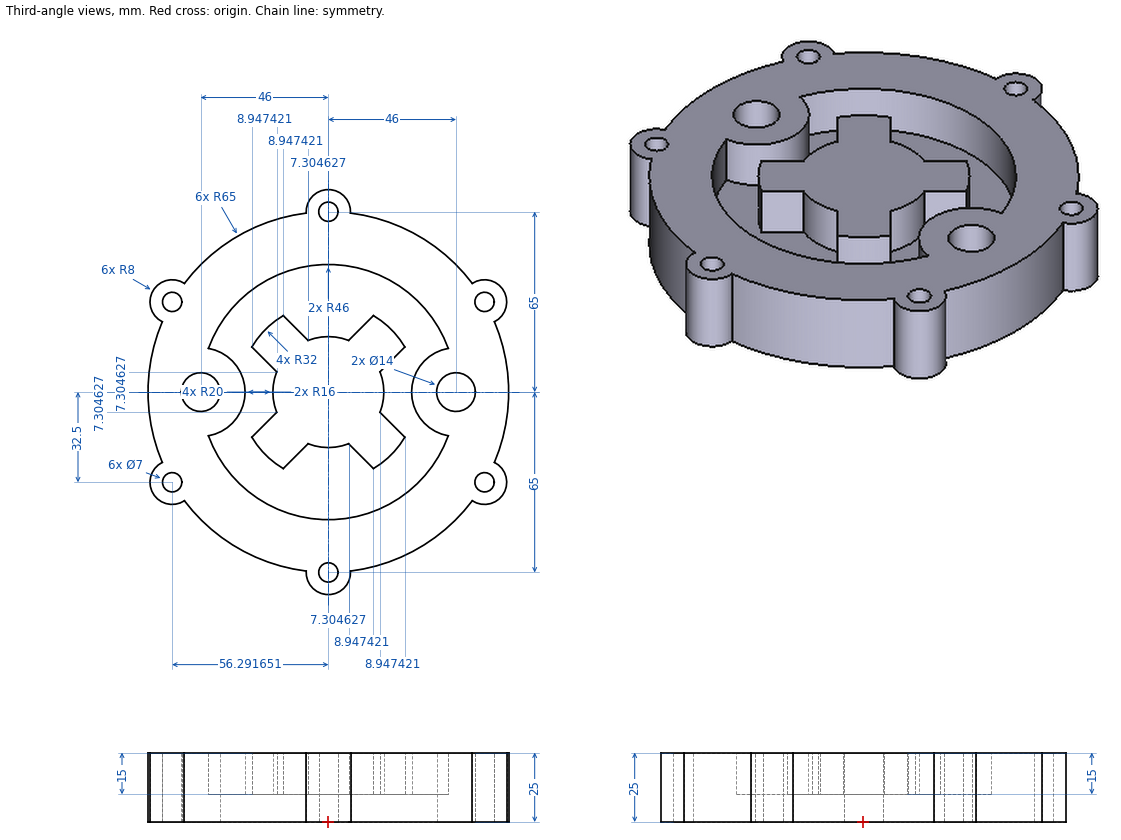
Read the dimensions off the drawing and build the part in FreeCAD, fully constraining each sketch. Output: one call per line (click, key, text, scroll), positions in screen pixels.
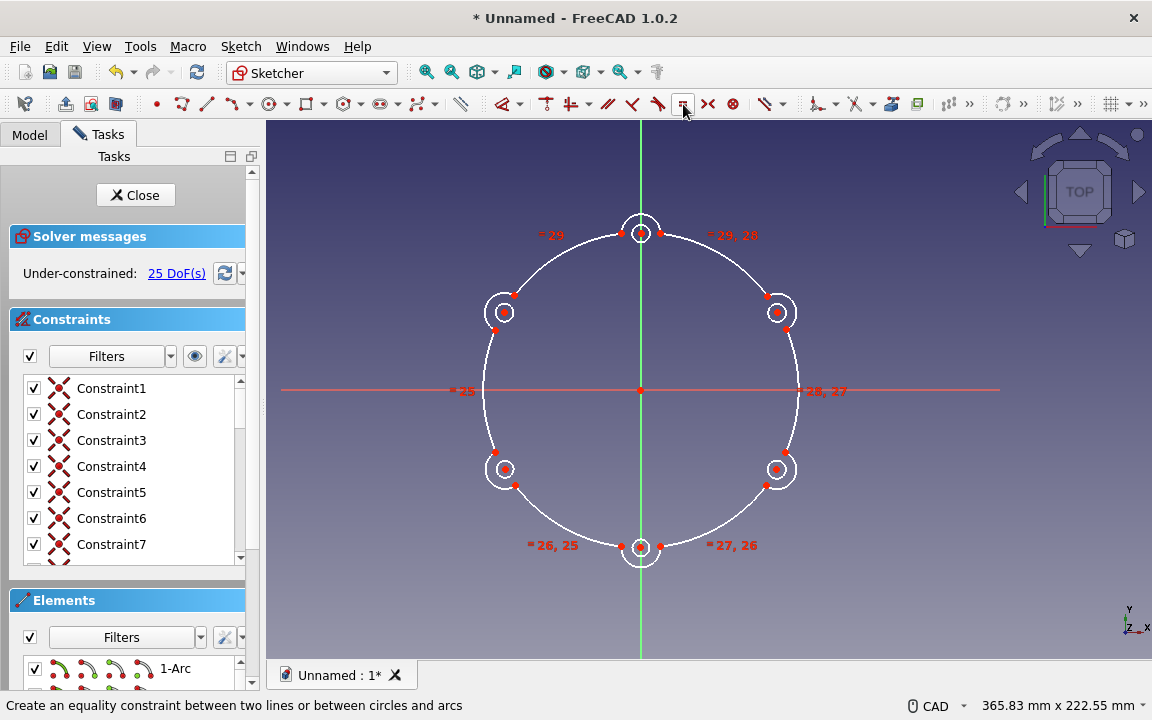
scroll(486, 467, up, 2)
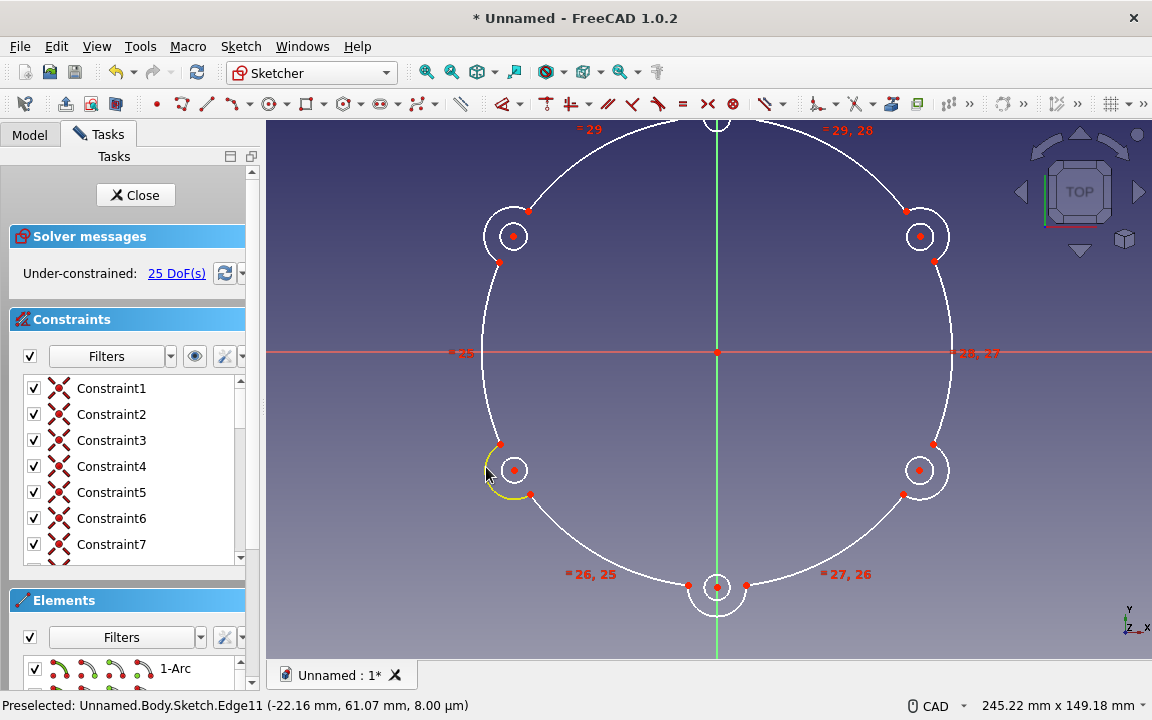
click(485, 467)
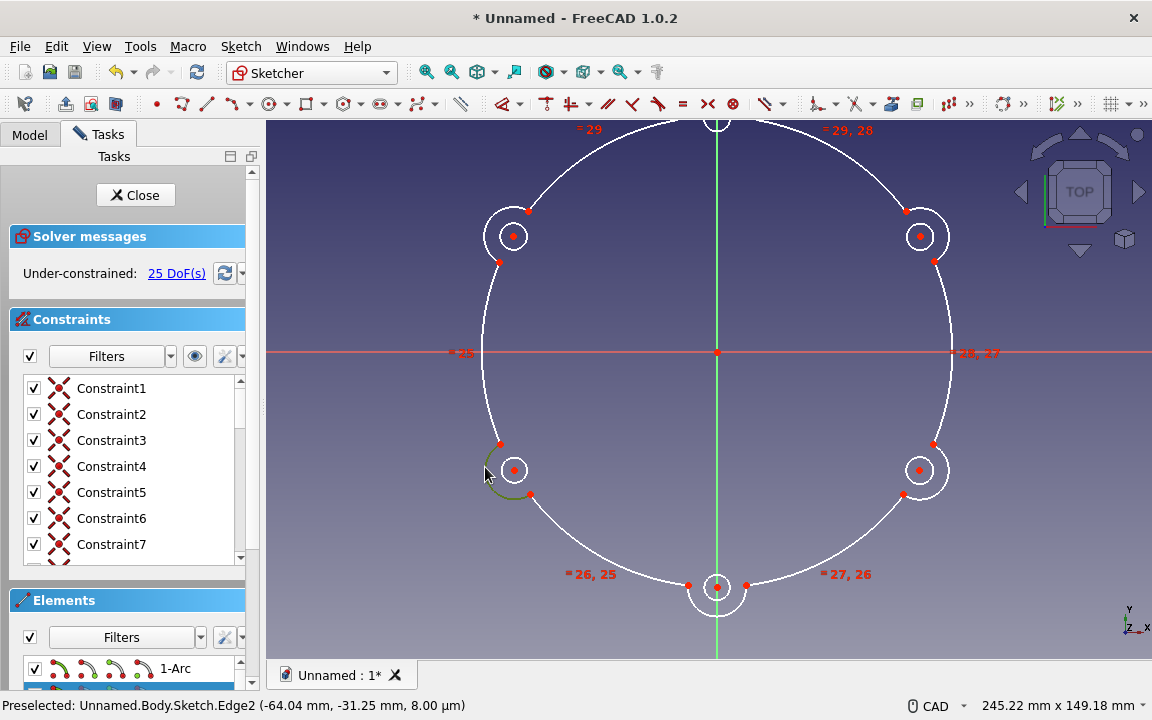
click(699, 611)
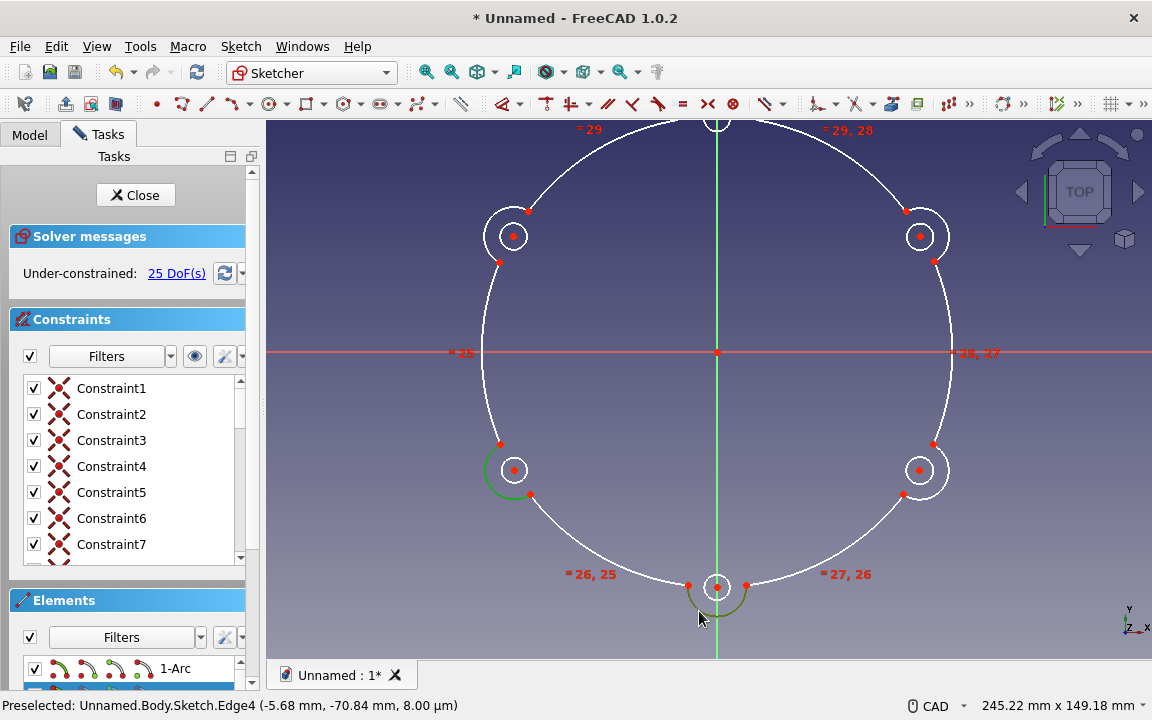
click(931, 497)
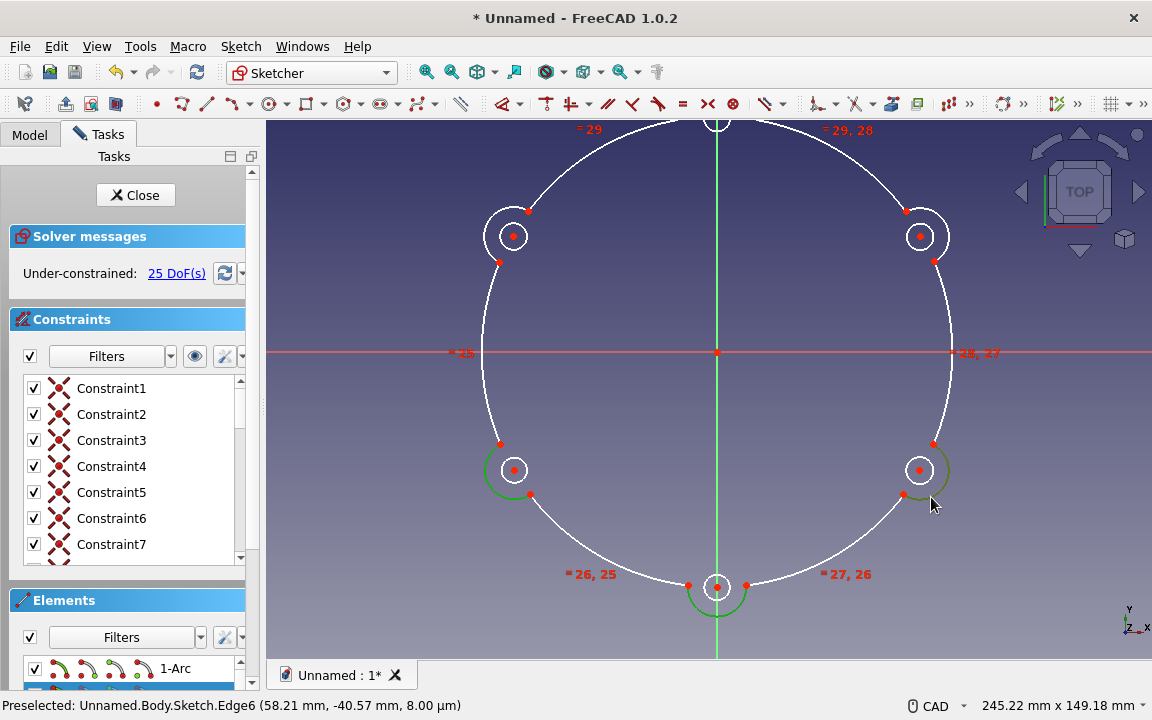
click(949, 240)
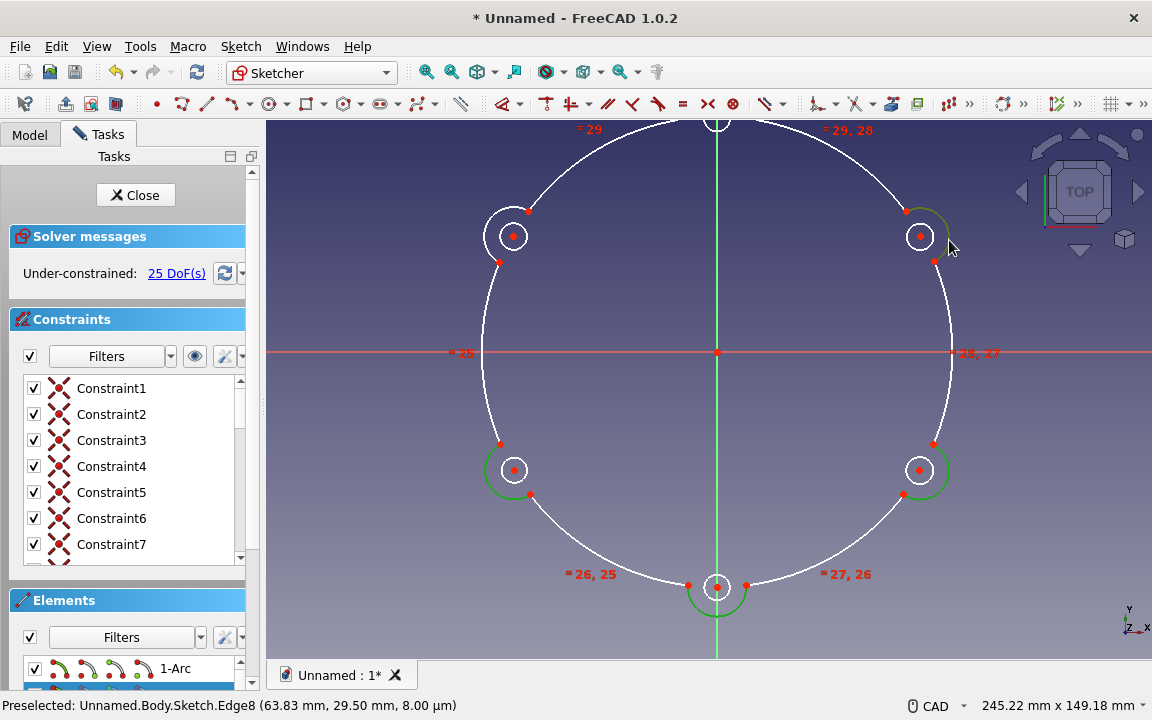
scroll(485, 466, down, 2)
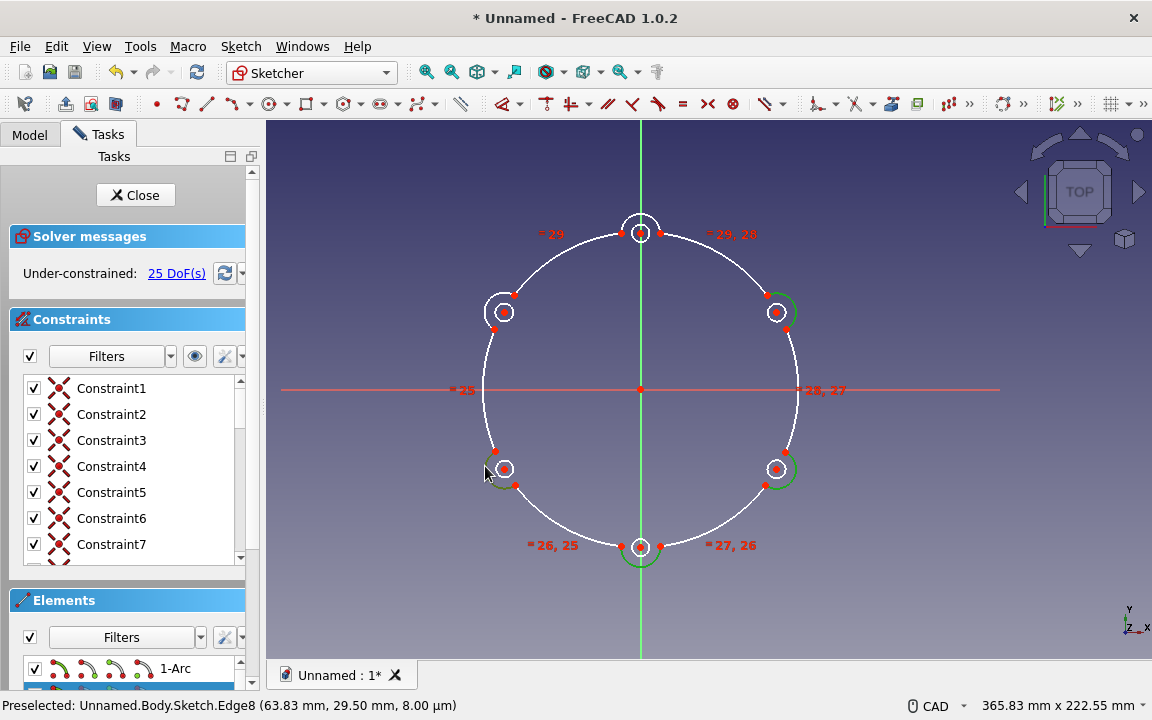
scroll(652, 218, up, 2)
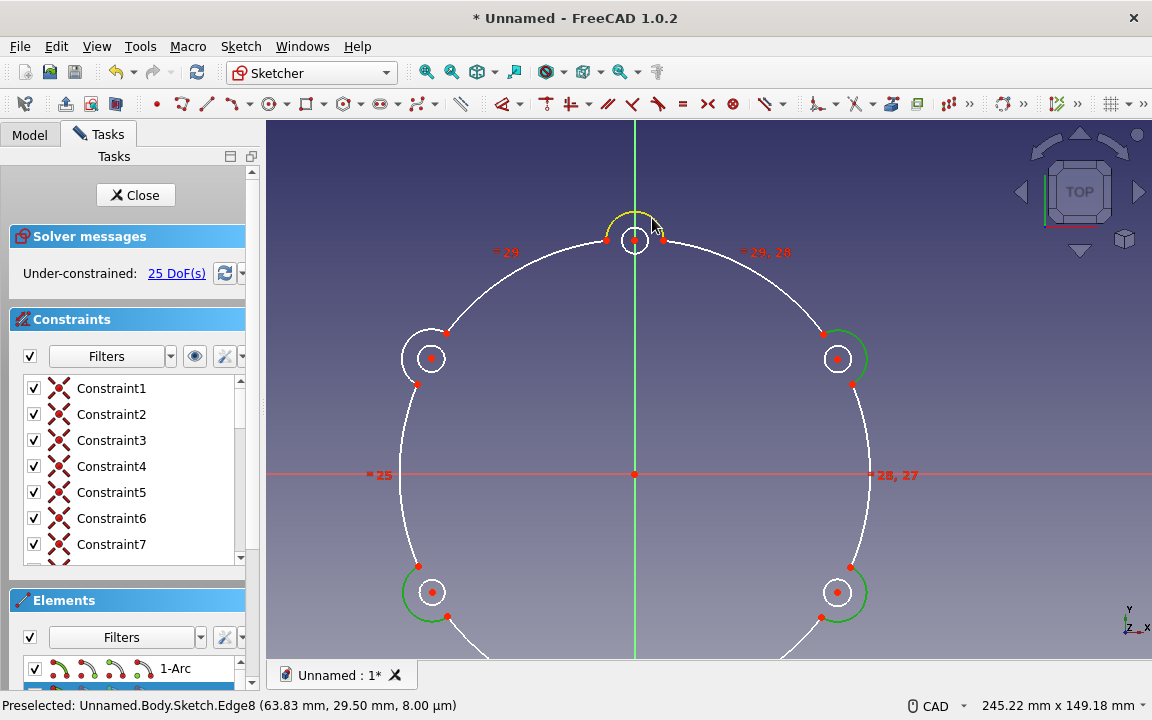
click(652, 217)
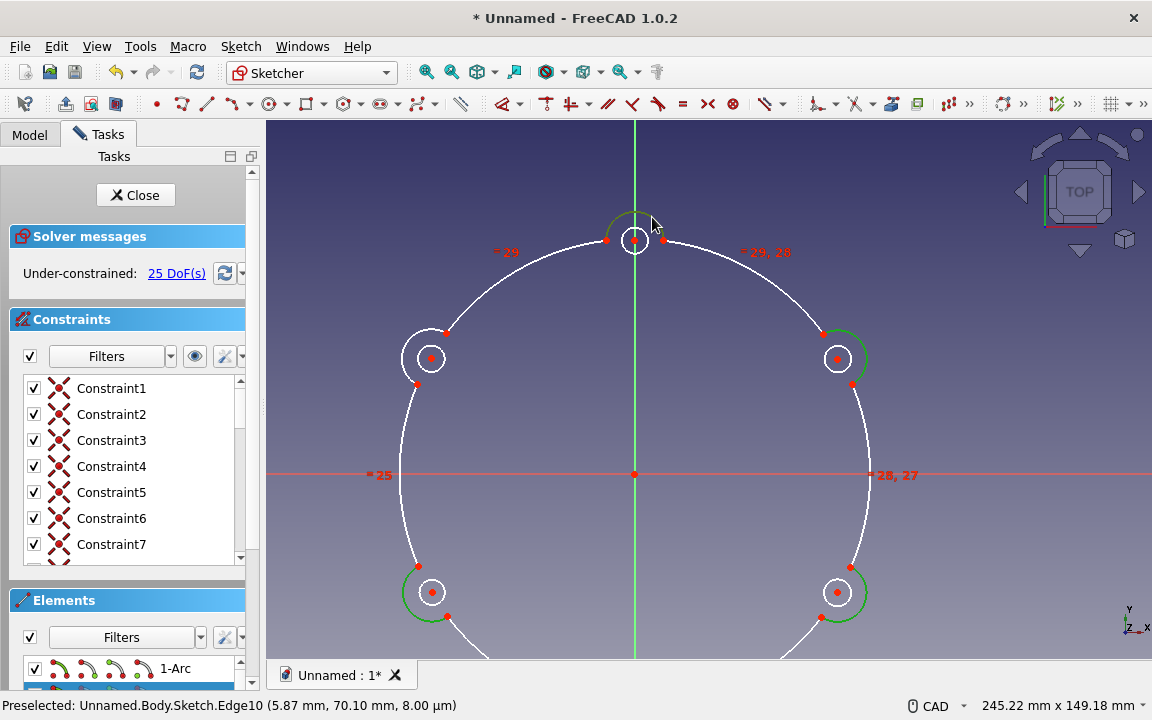
click(419, 332)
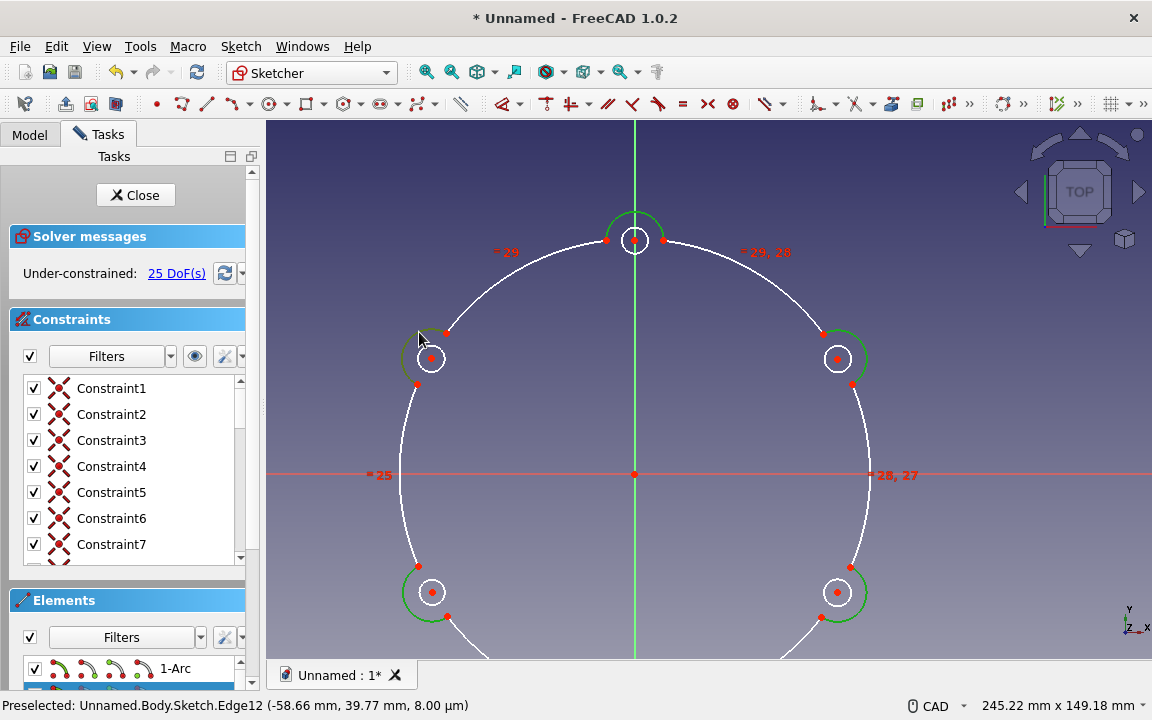
click(683, 104)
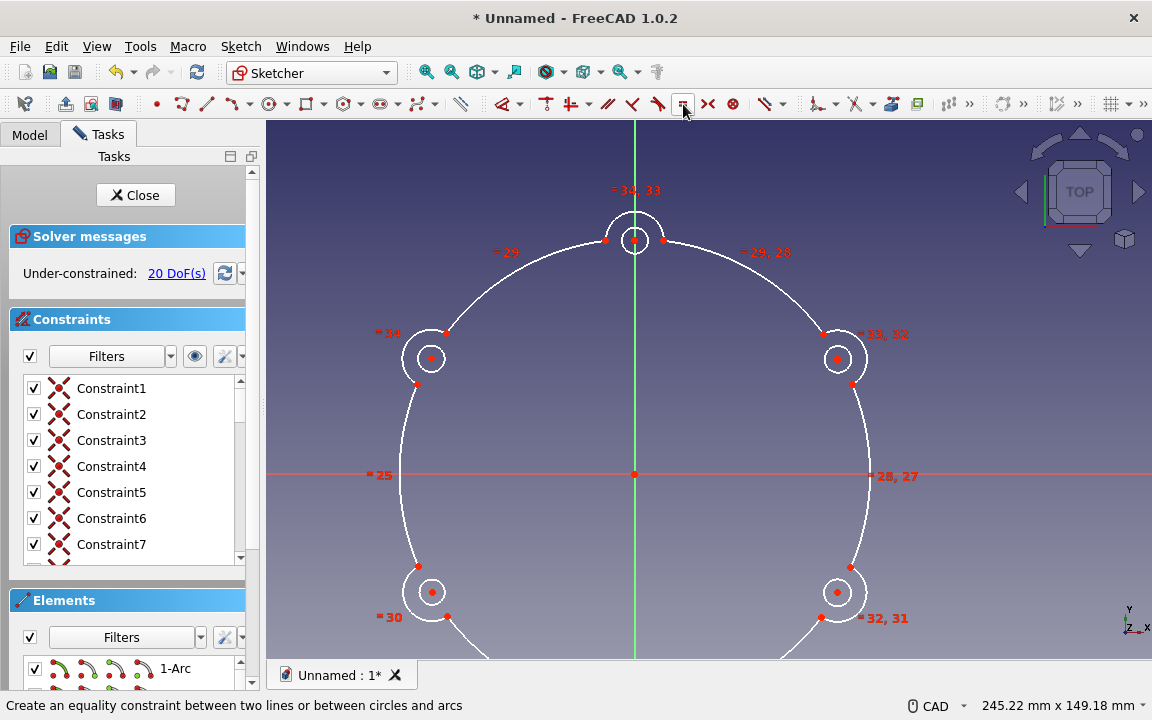
click(441, 583)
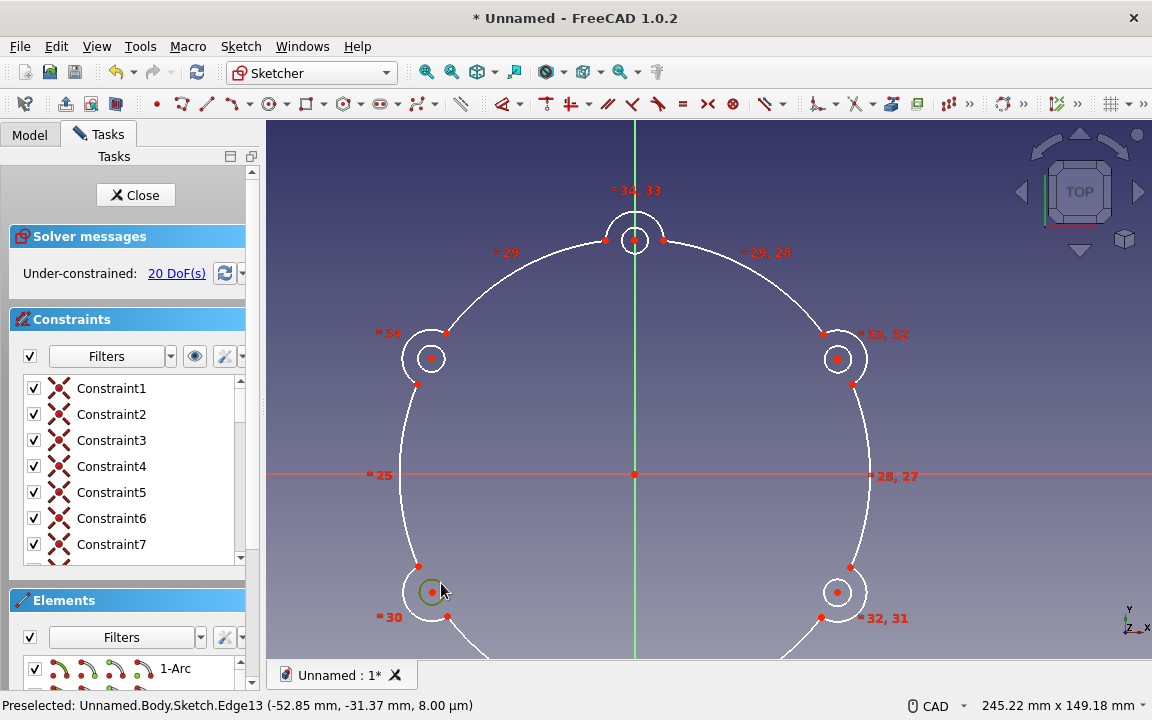
scroll(652, 217, down, 2)